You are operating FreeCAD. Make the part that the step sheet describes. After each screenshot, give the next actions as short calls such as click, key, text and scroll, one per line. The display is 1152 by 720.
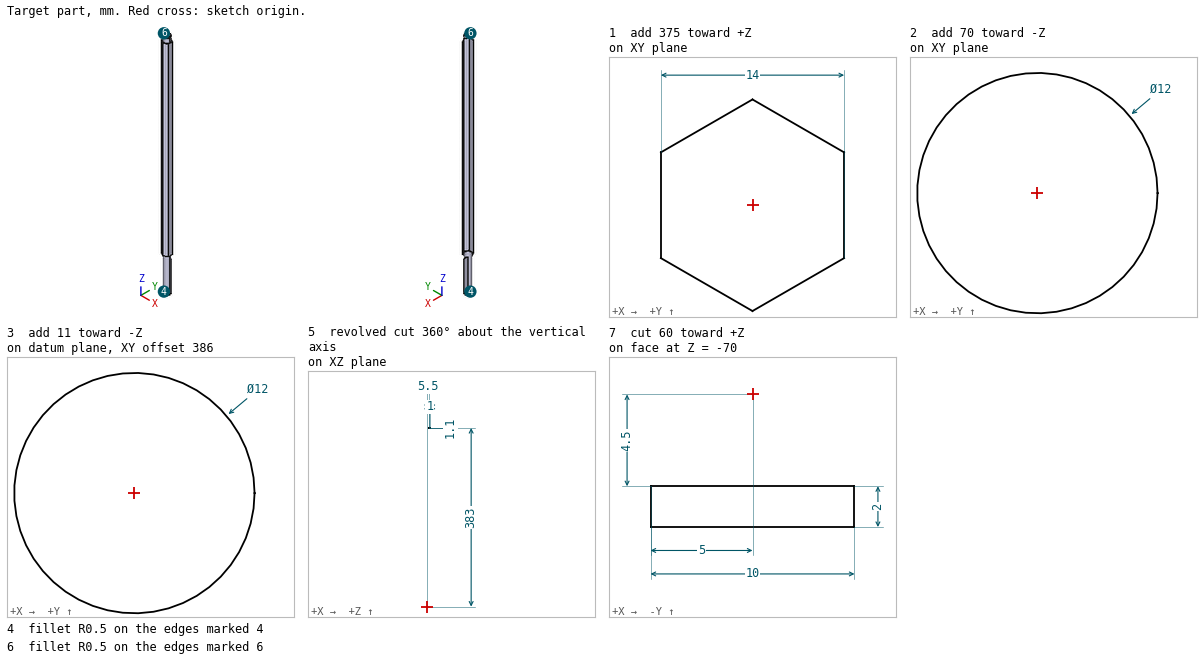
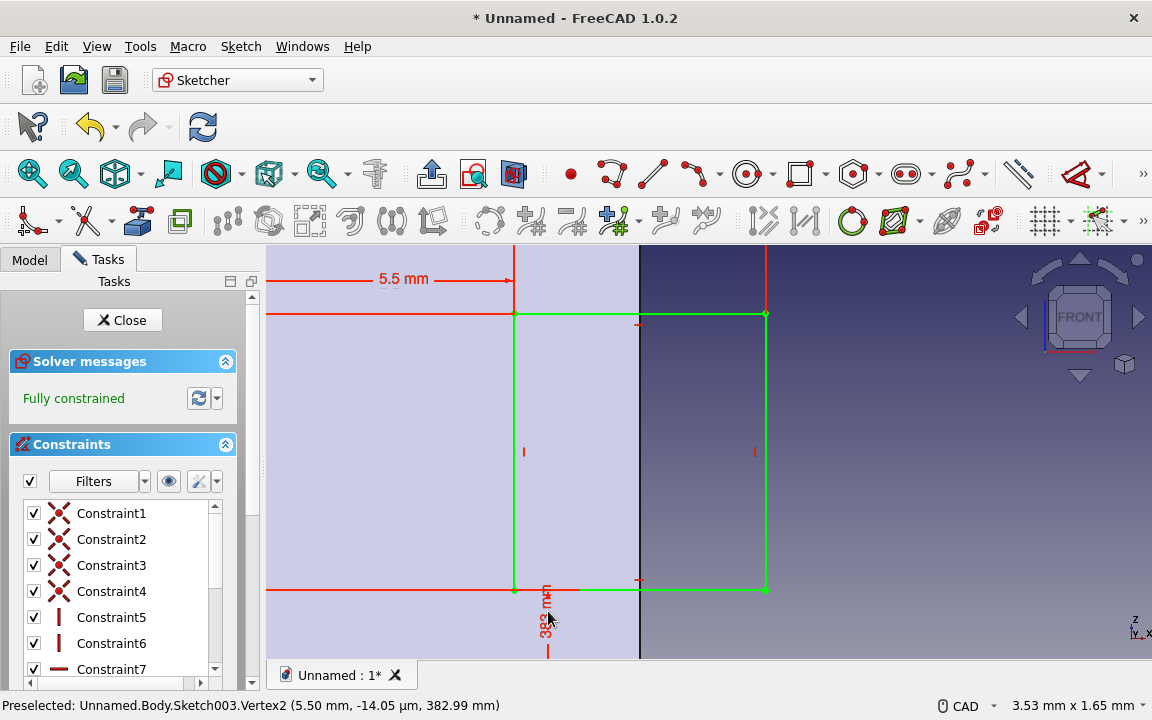
click(123, 320)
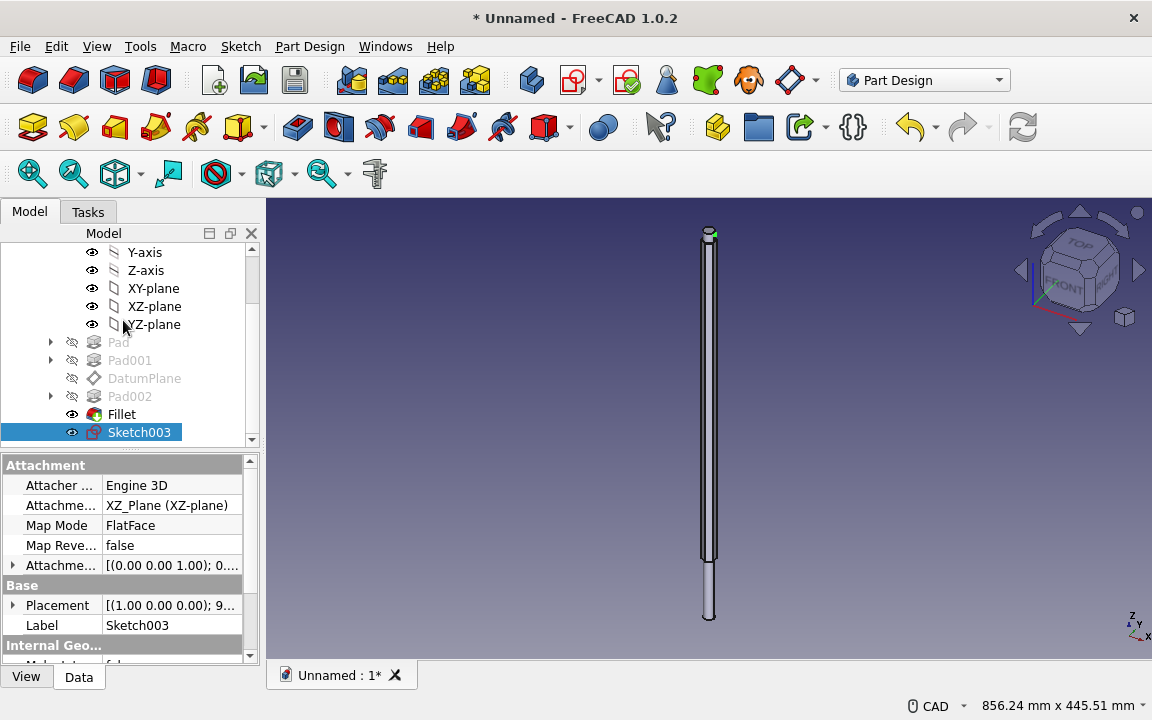
click(380, 128)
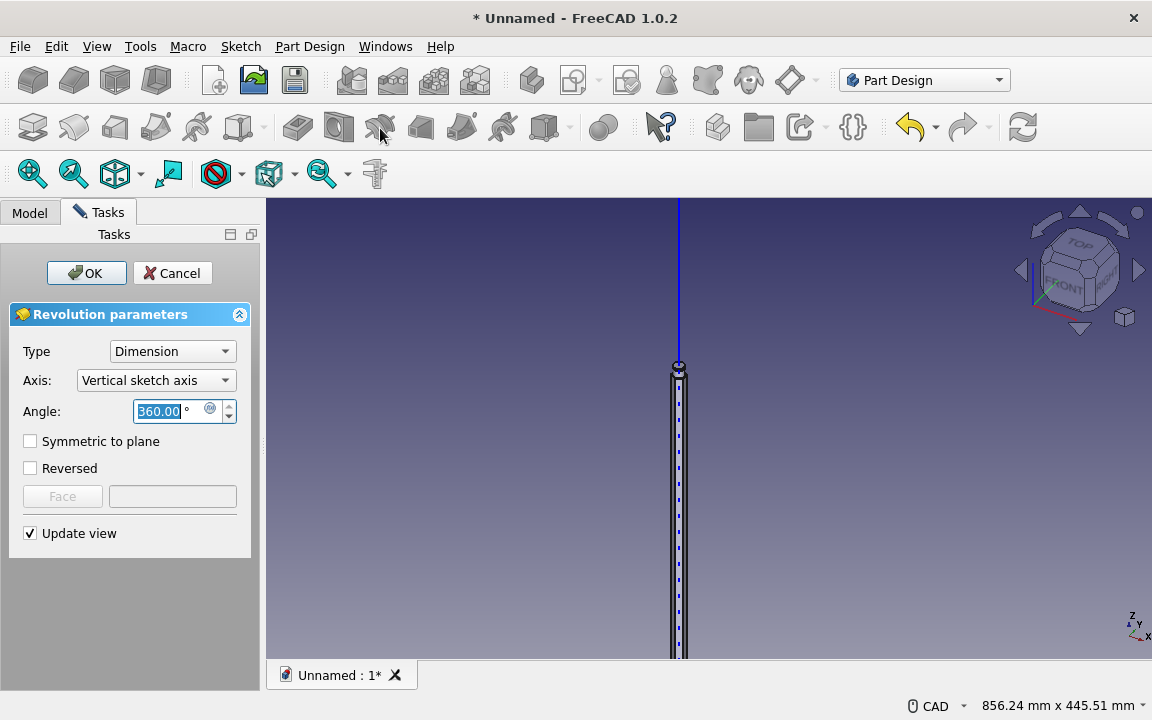
click(87, 273)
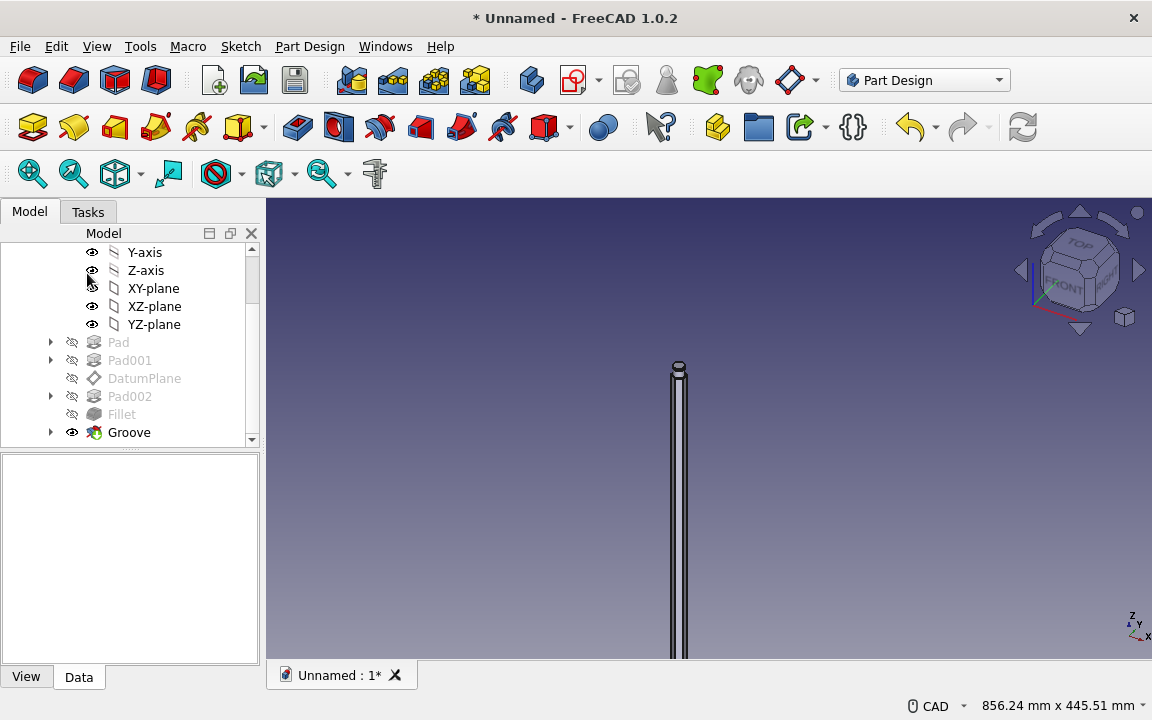
click(33, 174)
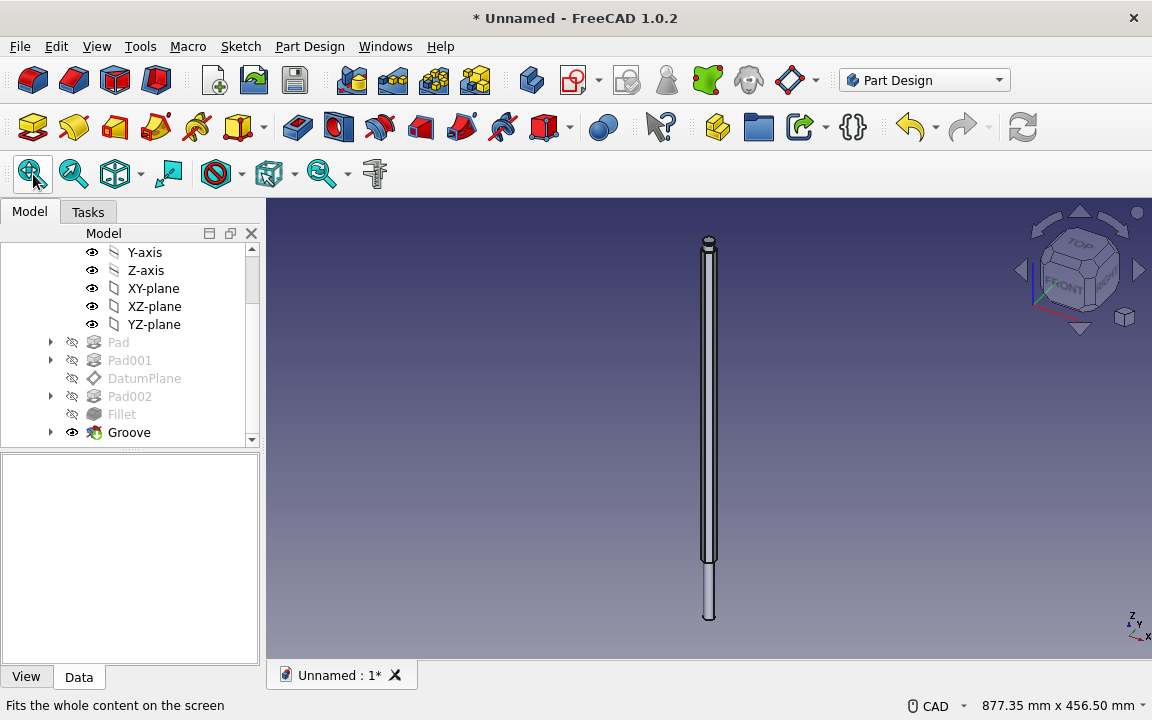
click(704, 237)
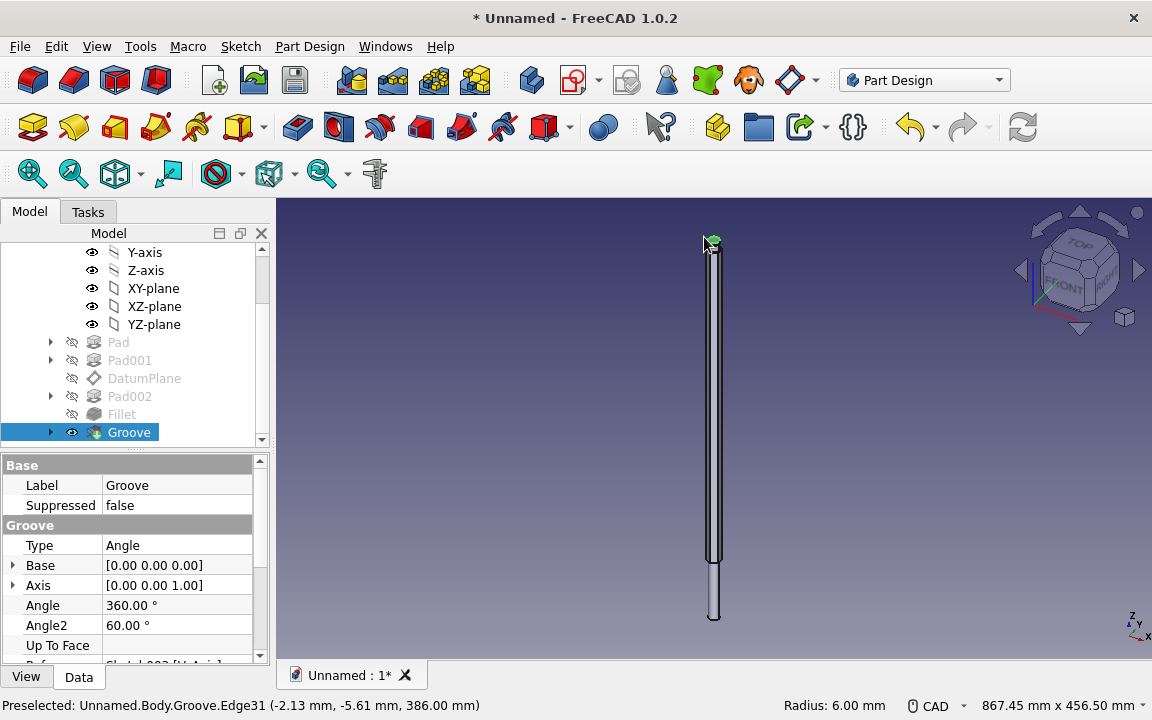
click(33, 80)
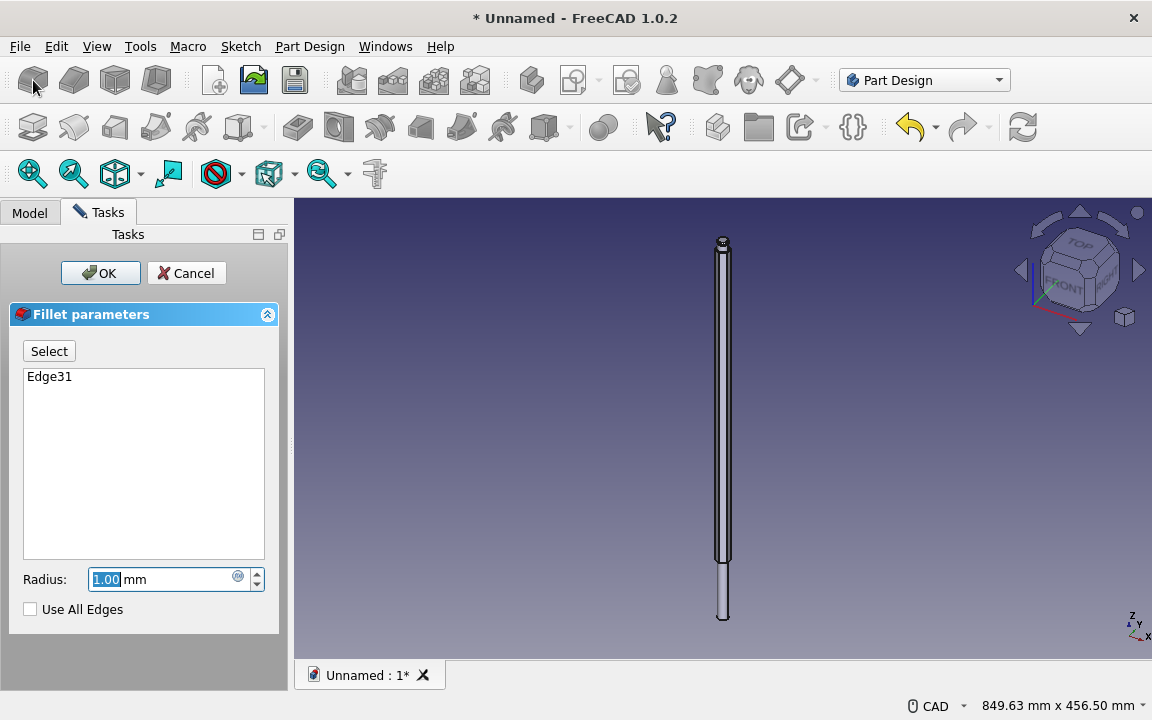
text(0.5)
key(Tab)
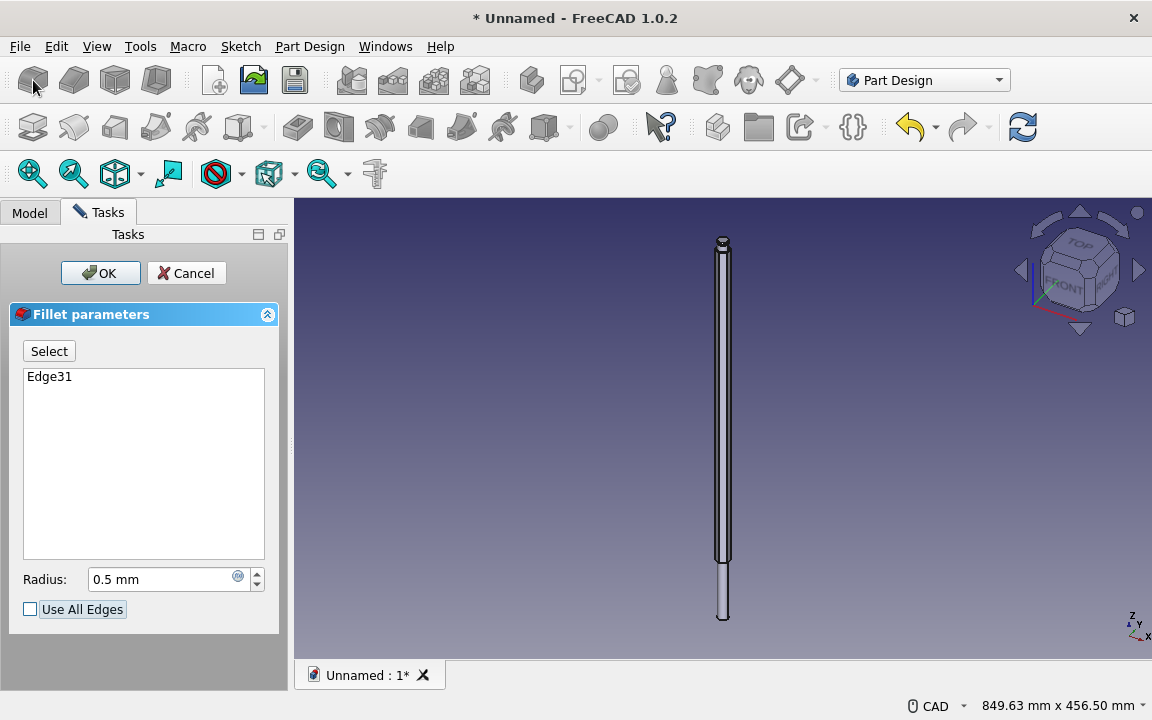
click(101, 273)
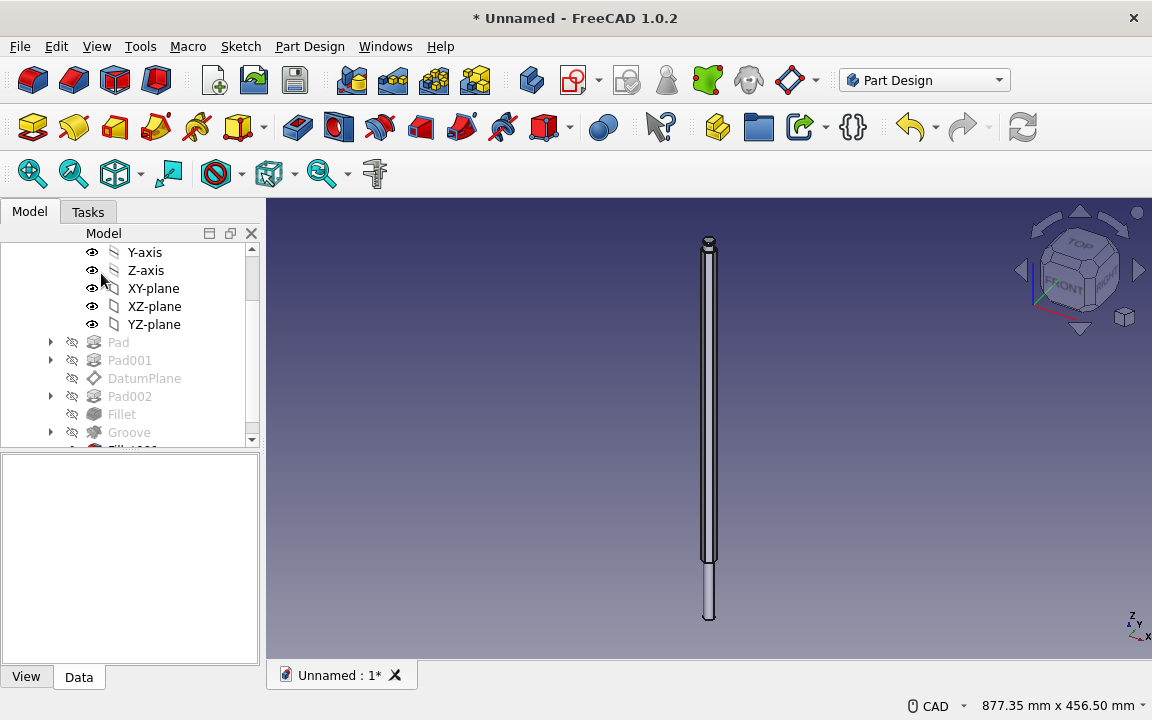
key(5)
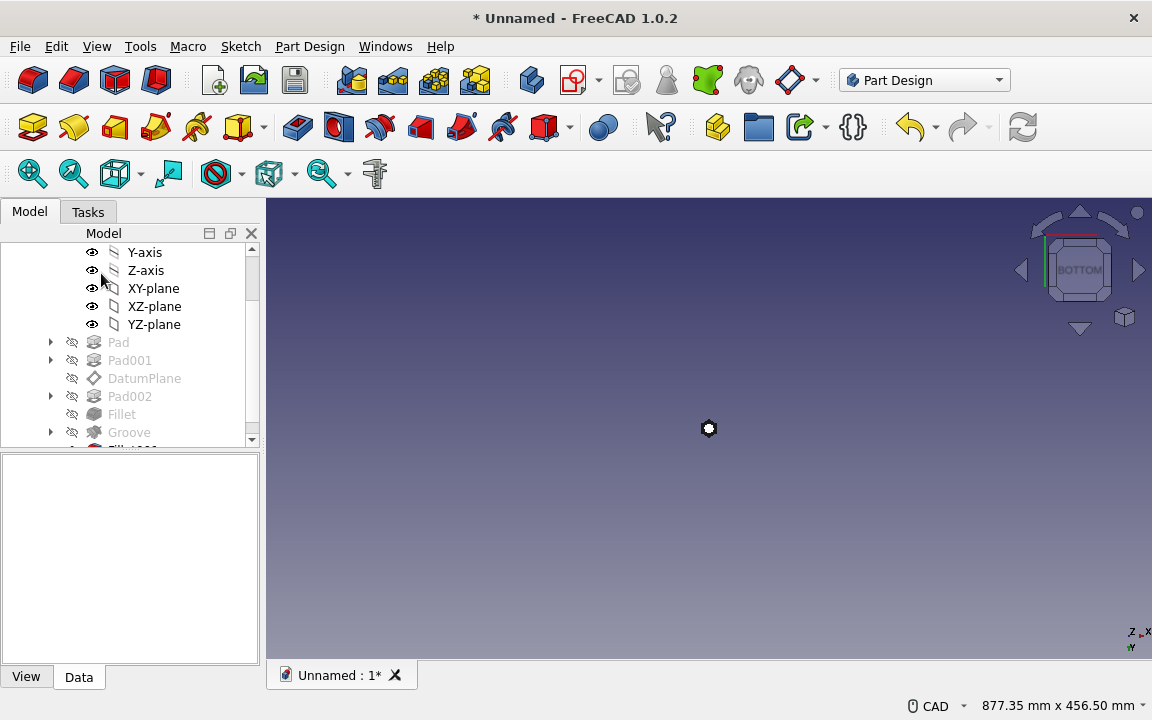
click(33, 174)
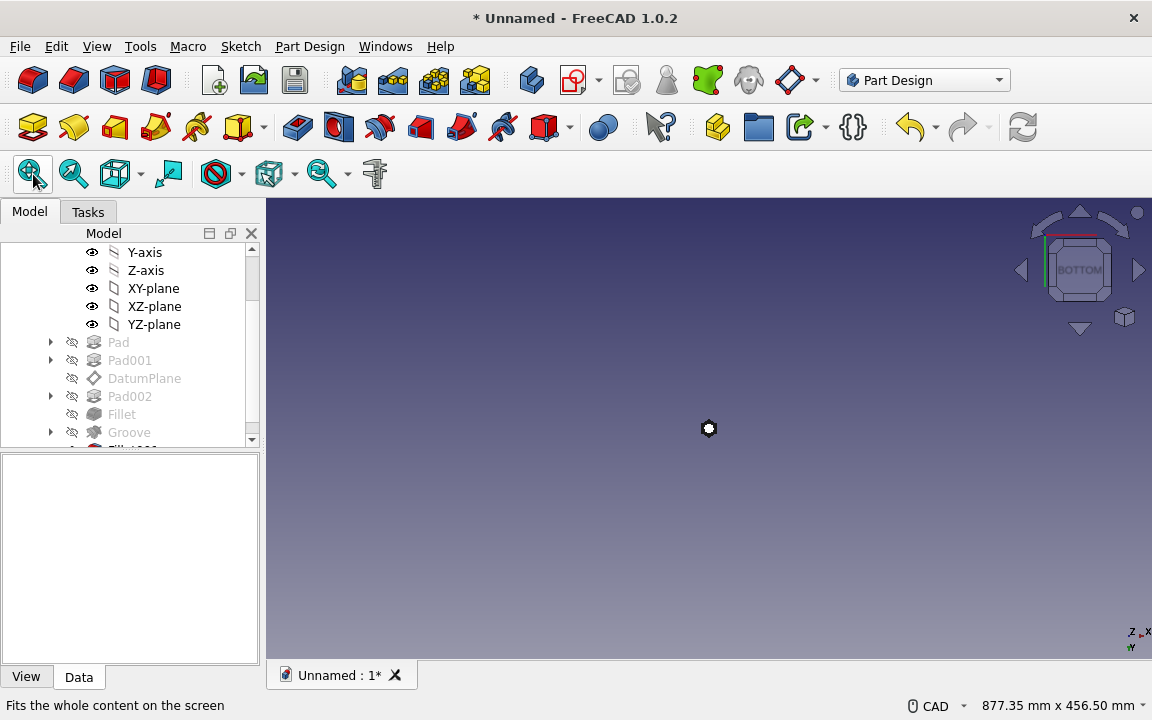
scroll(709, 427, up, 4)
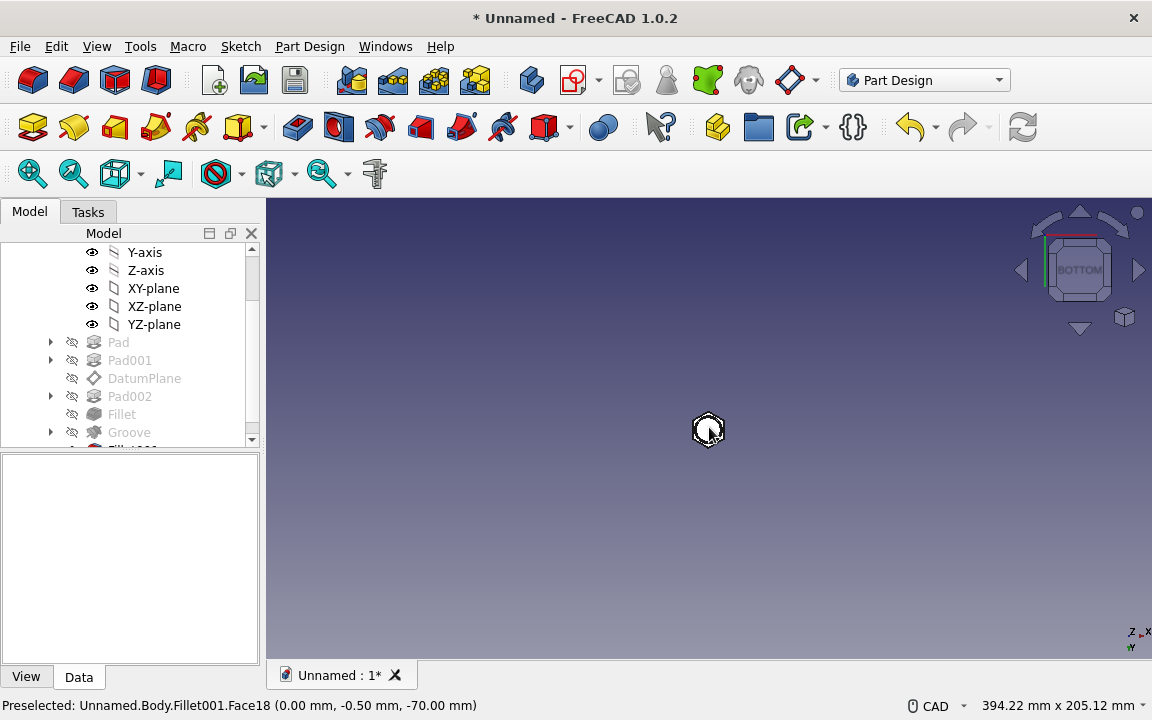
click(708, 429)